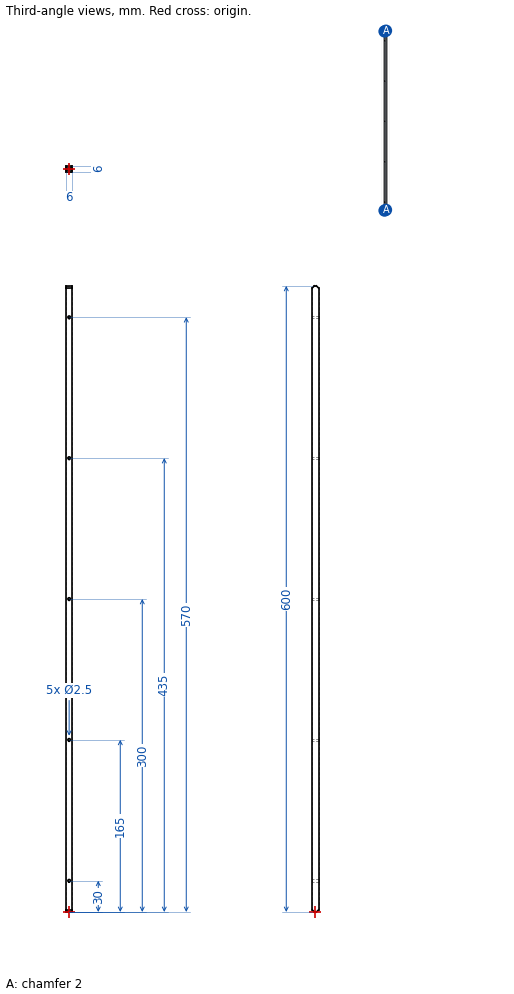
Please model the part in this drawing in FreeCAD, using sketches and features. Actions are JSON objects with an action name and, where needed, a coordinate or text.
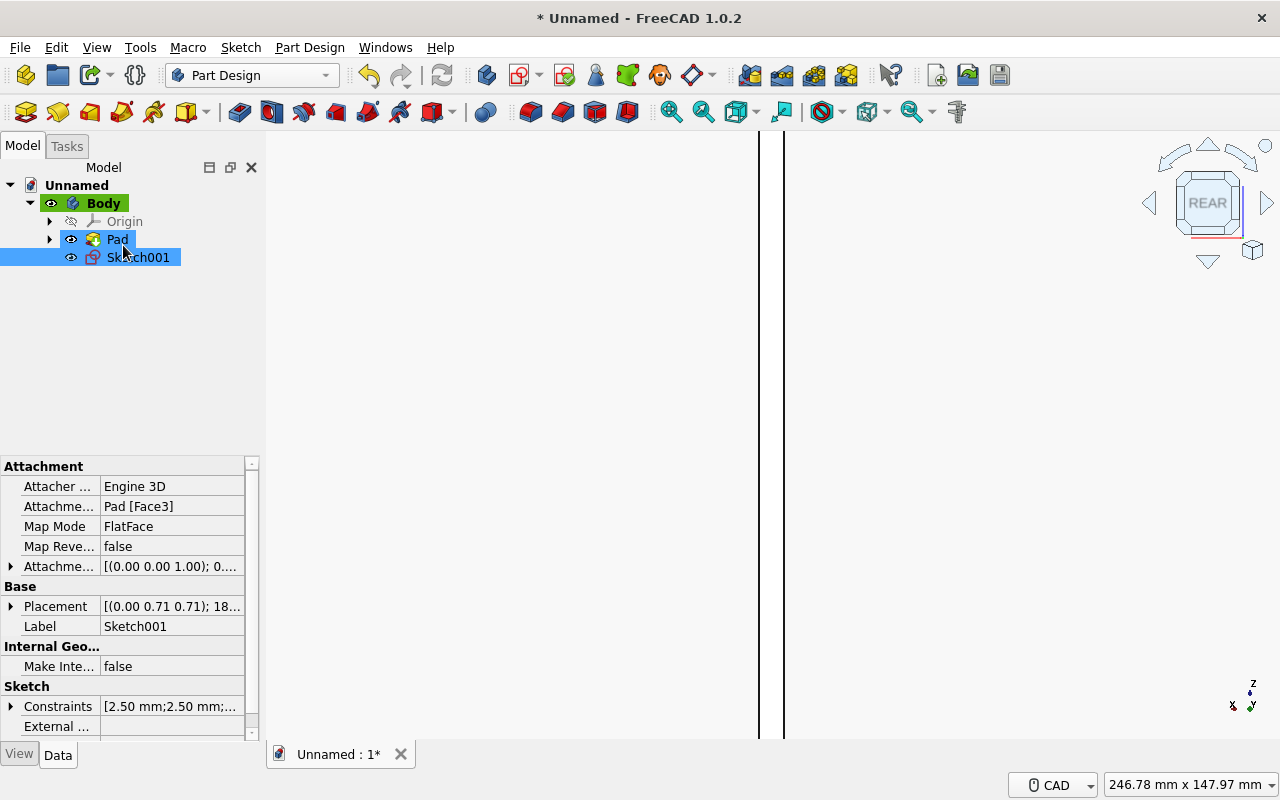
{"action": "left_click", "coordinate": [240, 112]}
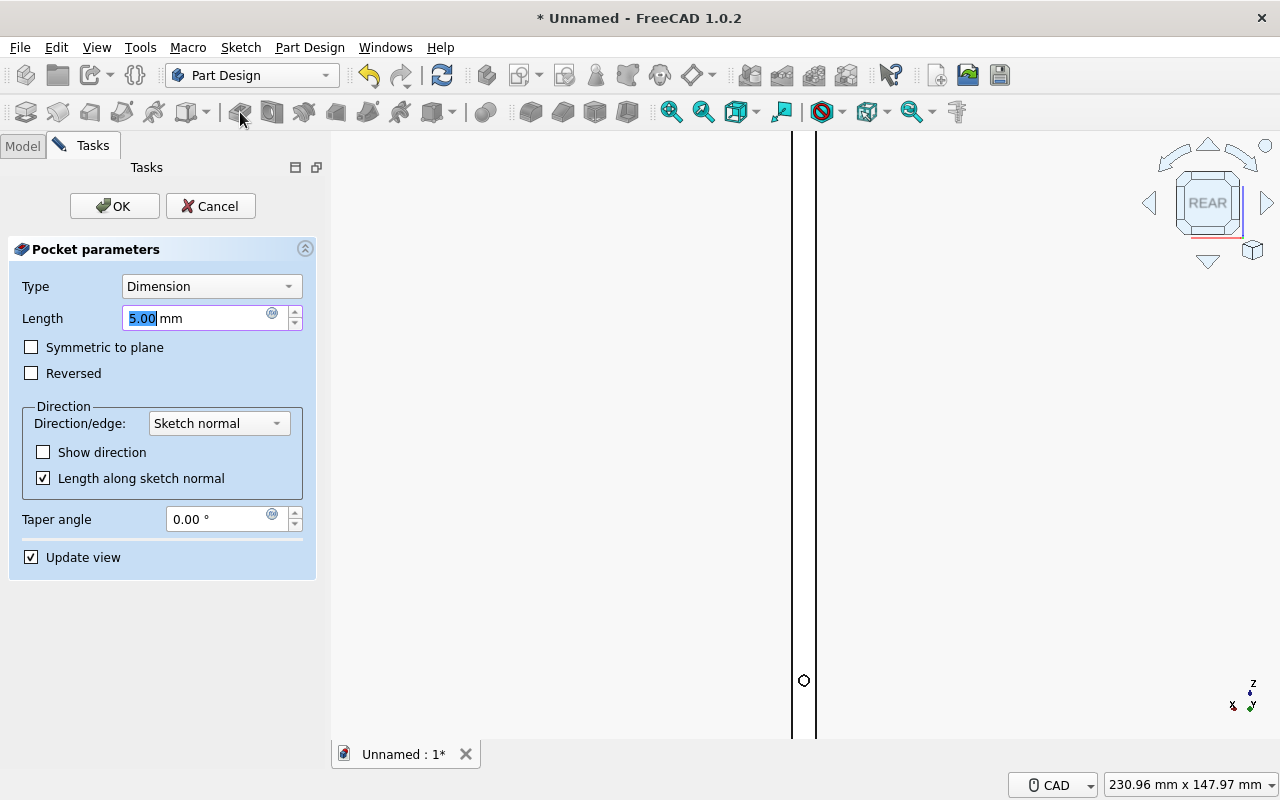
{"action": "left_click", "coordinate": [212, 286]}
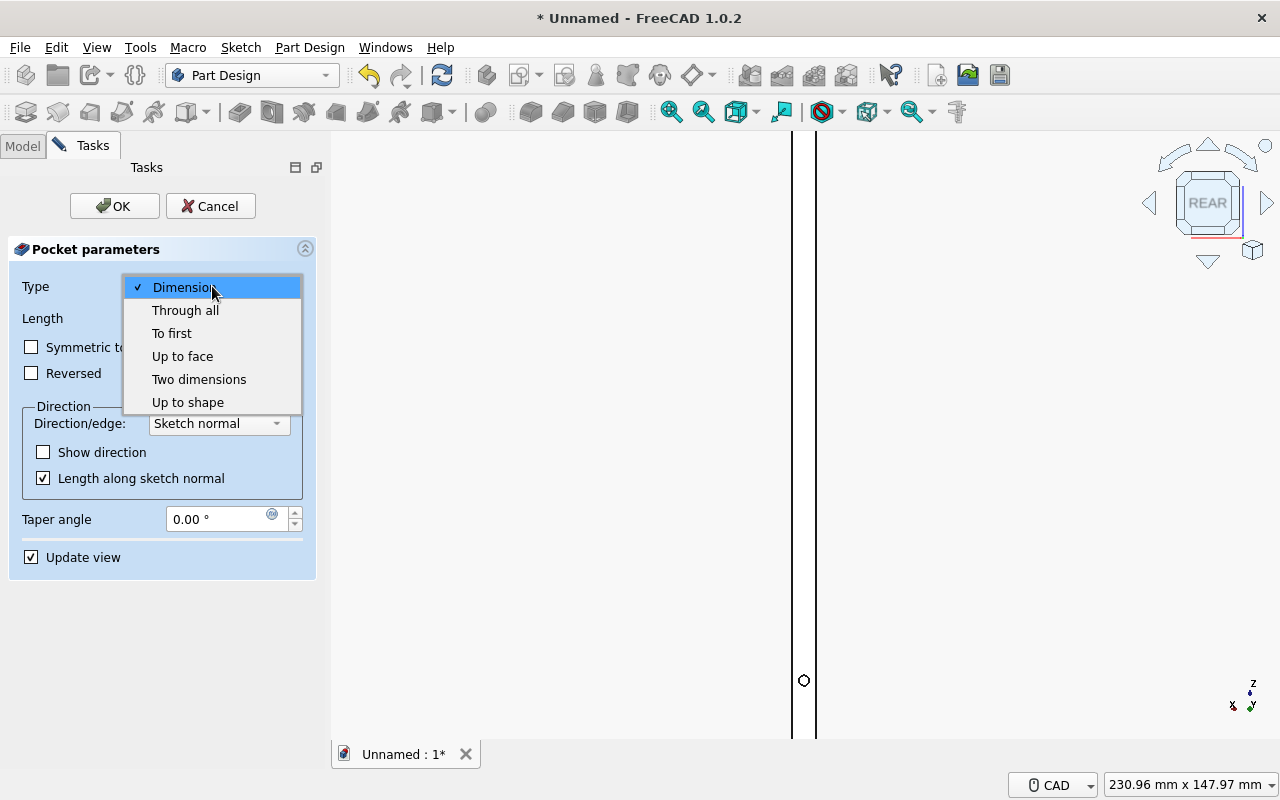
{"action": "left_click", "coordinate": [212, 310]}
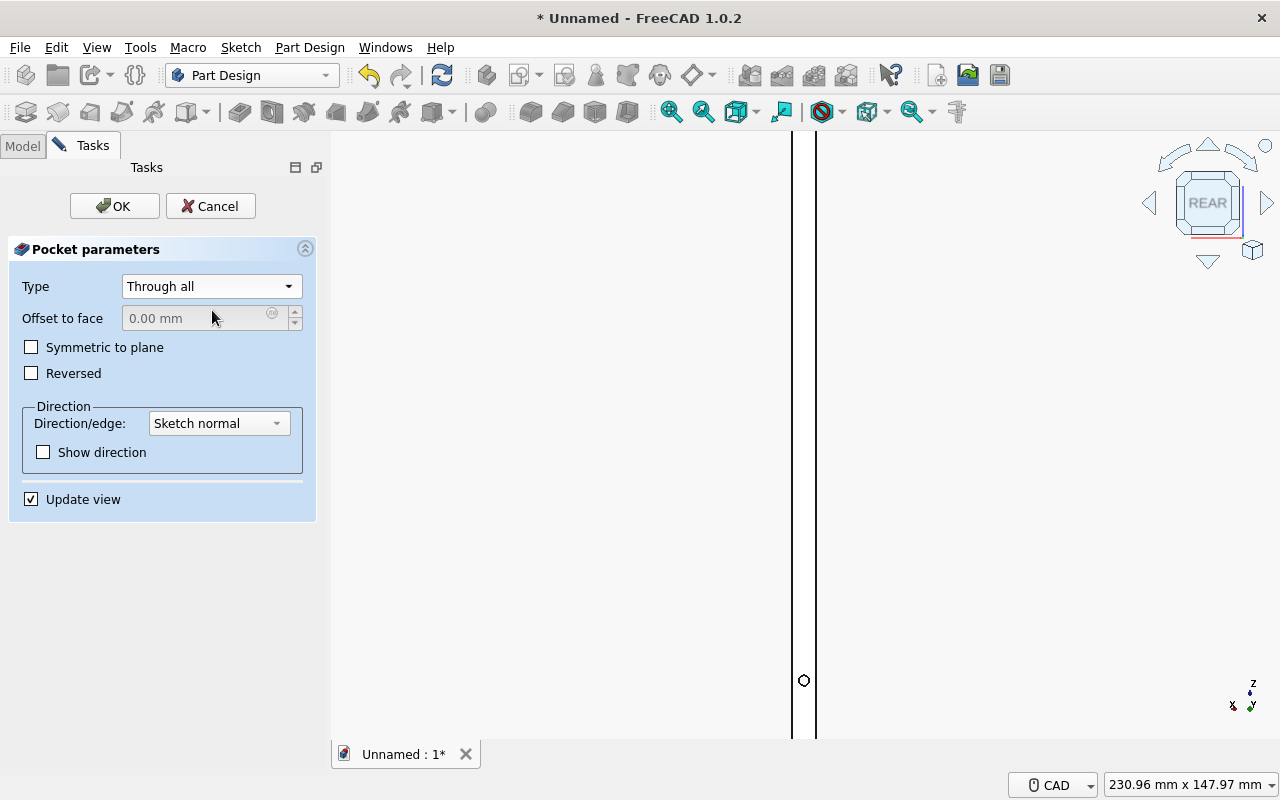
{"action": "left_click", "coordinate": [115, 206]}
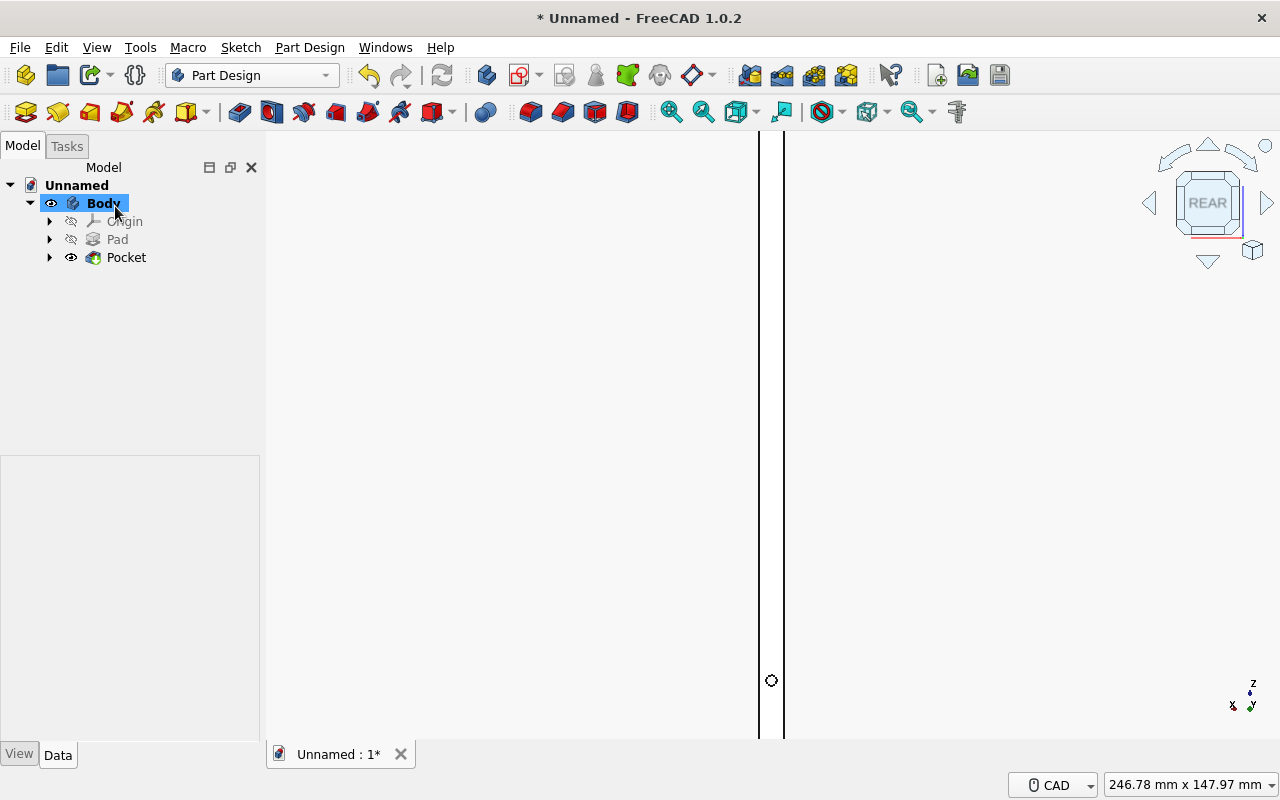
{"action": "left_click", "coordinate": [672, 112]}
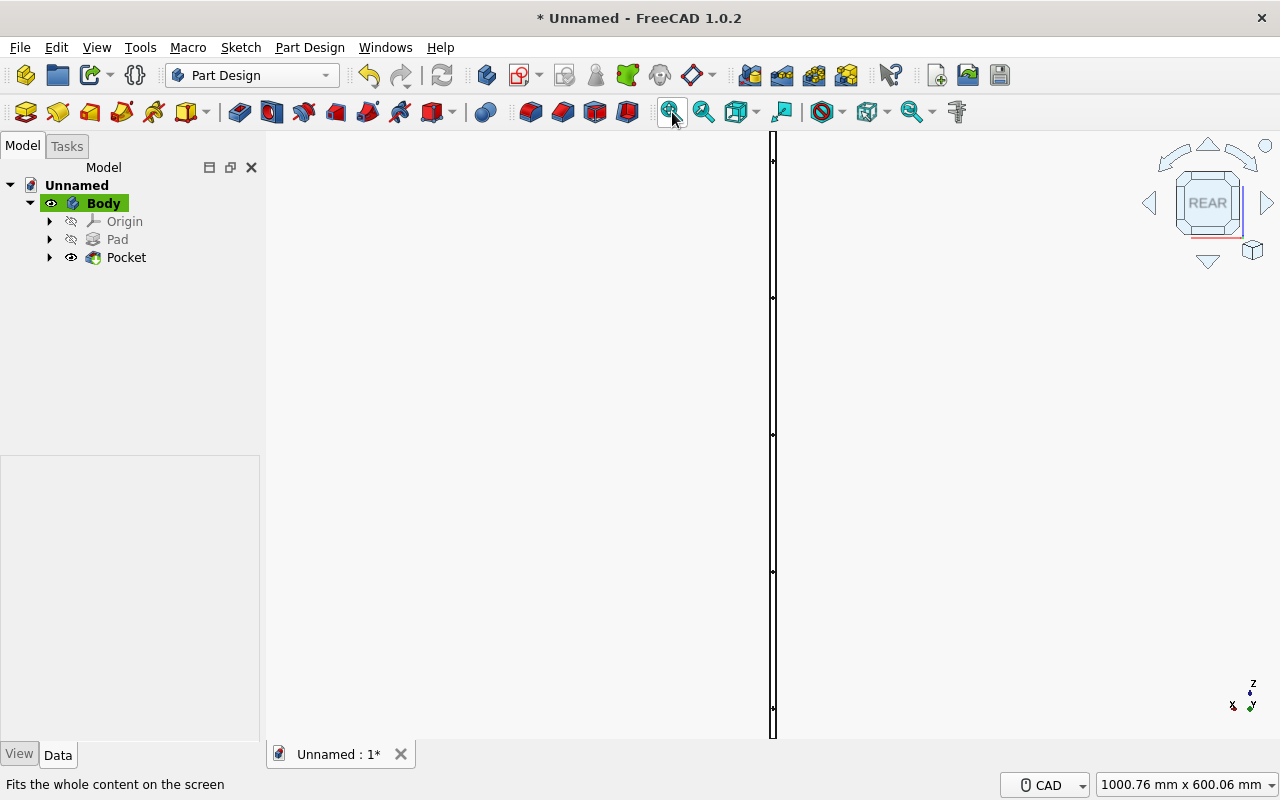
{"action": "key", "text": "0"}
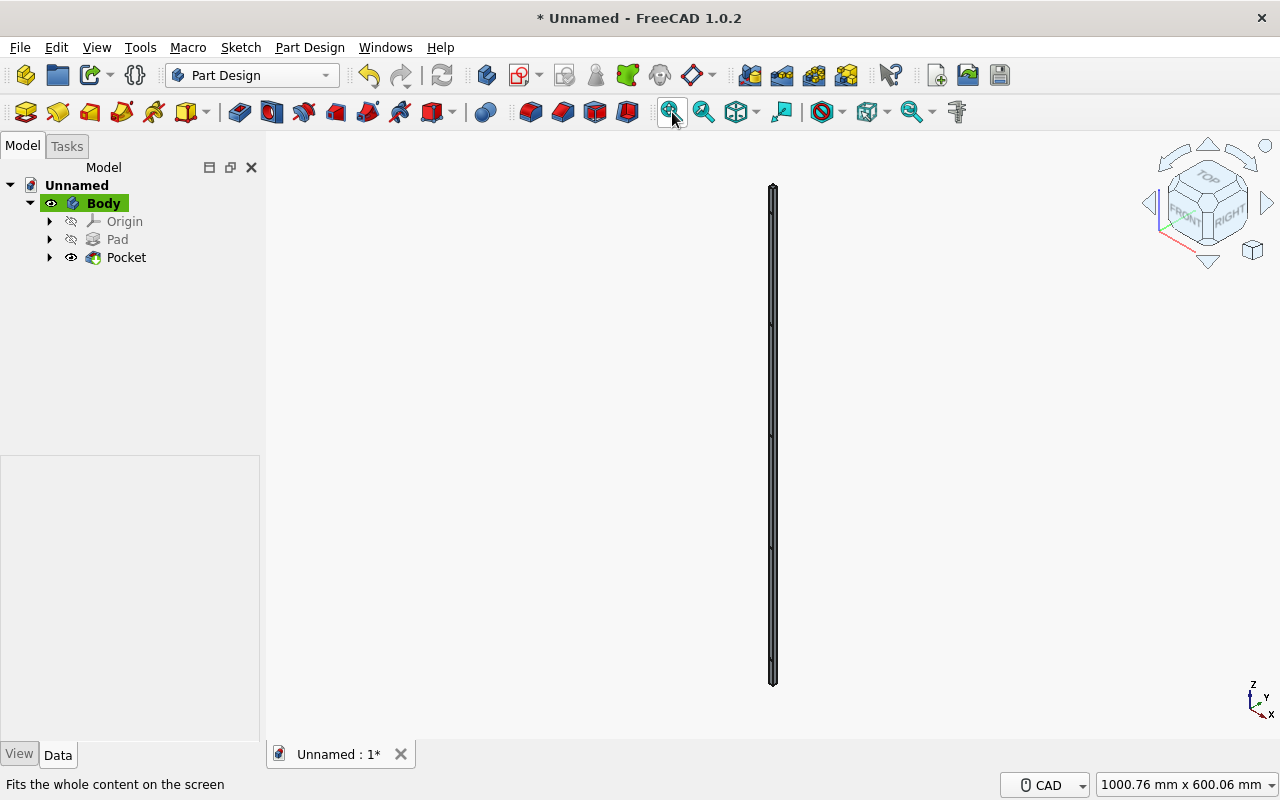
{"action": "scroll", "coordinate": [771, 187], "scroll_direction": "up", "scroll_amount": 10}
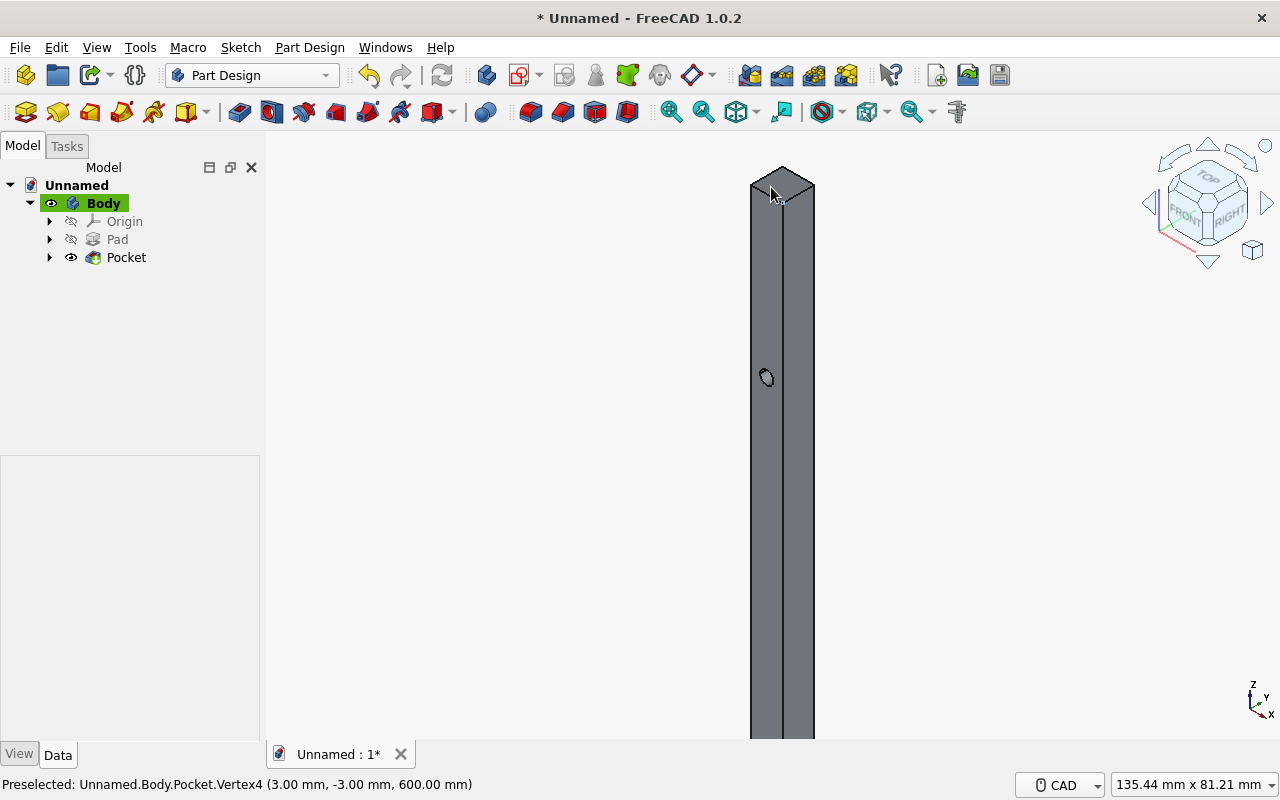
{"action": "left_click", "coordinate": [767, 193]}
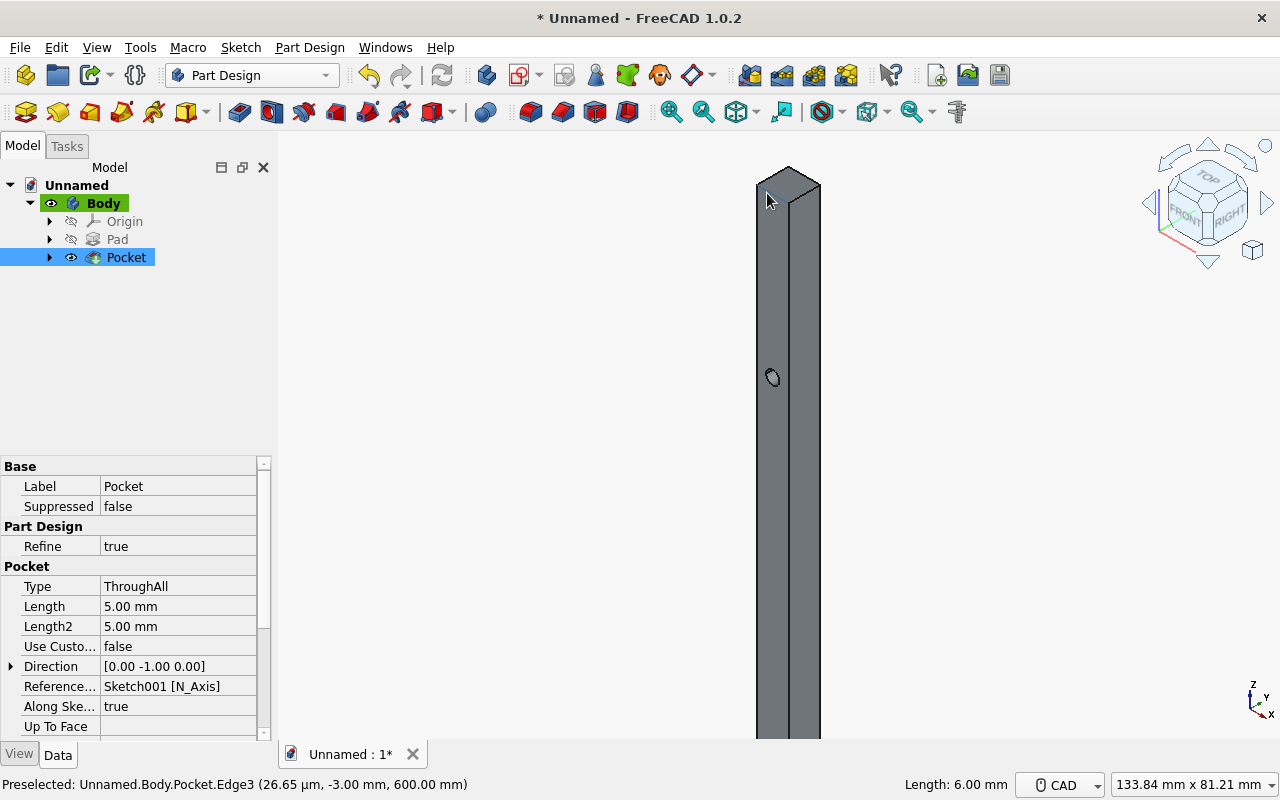
{"action": "left_click", "coordinate": [672, 112]}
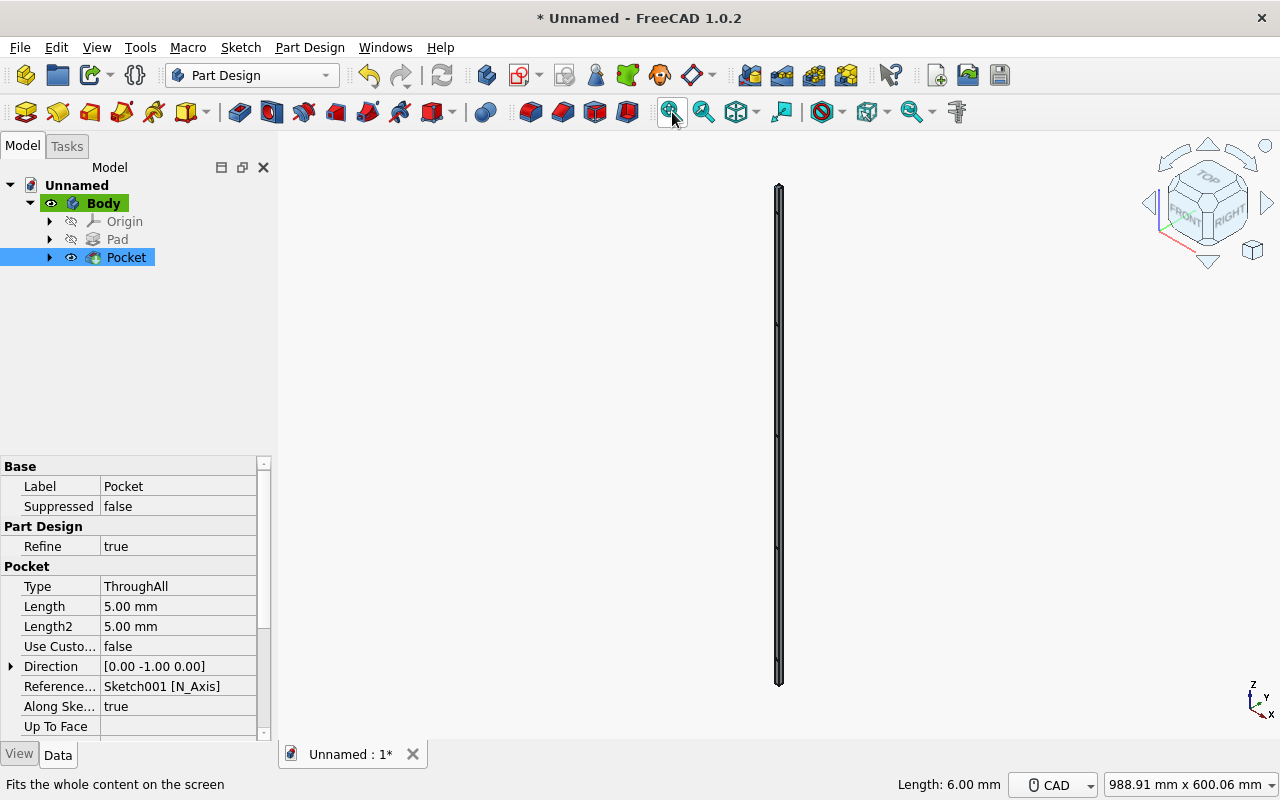
{"action": "key", "text": "2"}